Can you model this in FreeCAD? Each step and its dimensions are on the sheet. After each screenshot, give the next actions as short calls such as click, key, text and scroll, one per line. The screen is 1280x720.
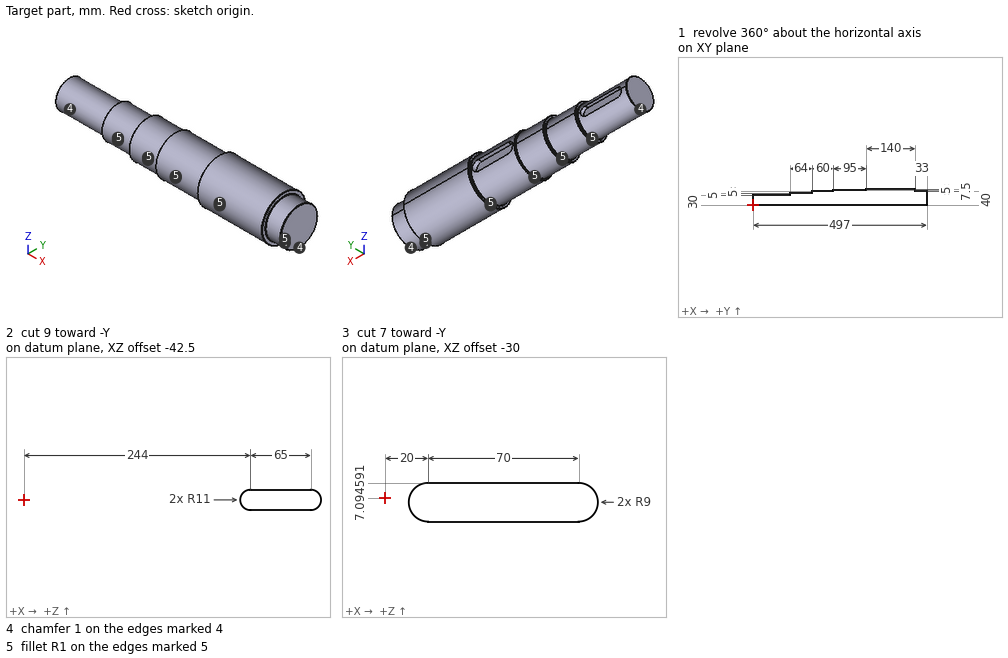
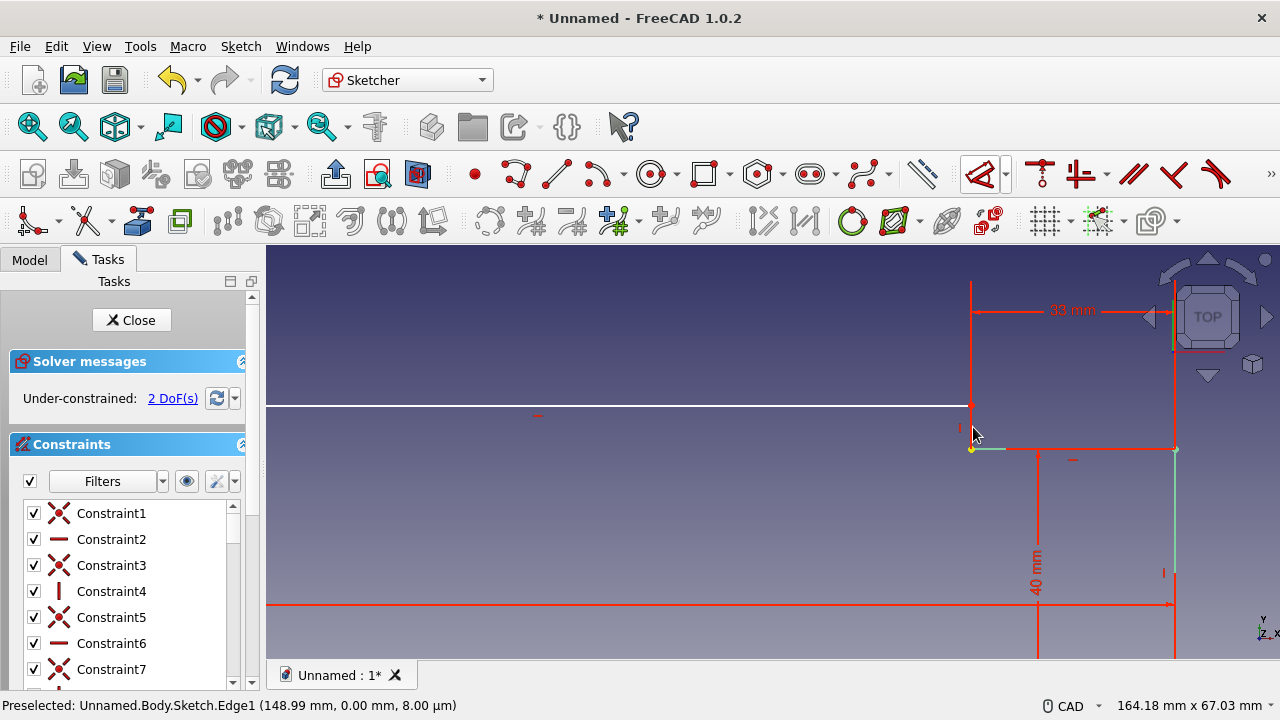
click(971, 427)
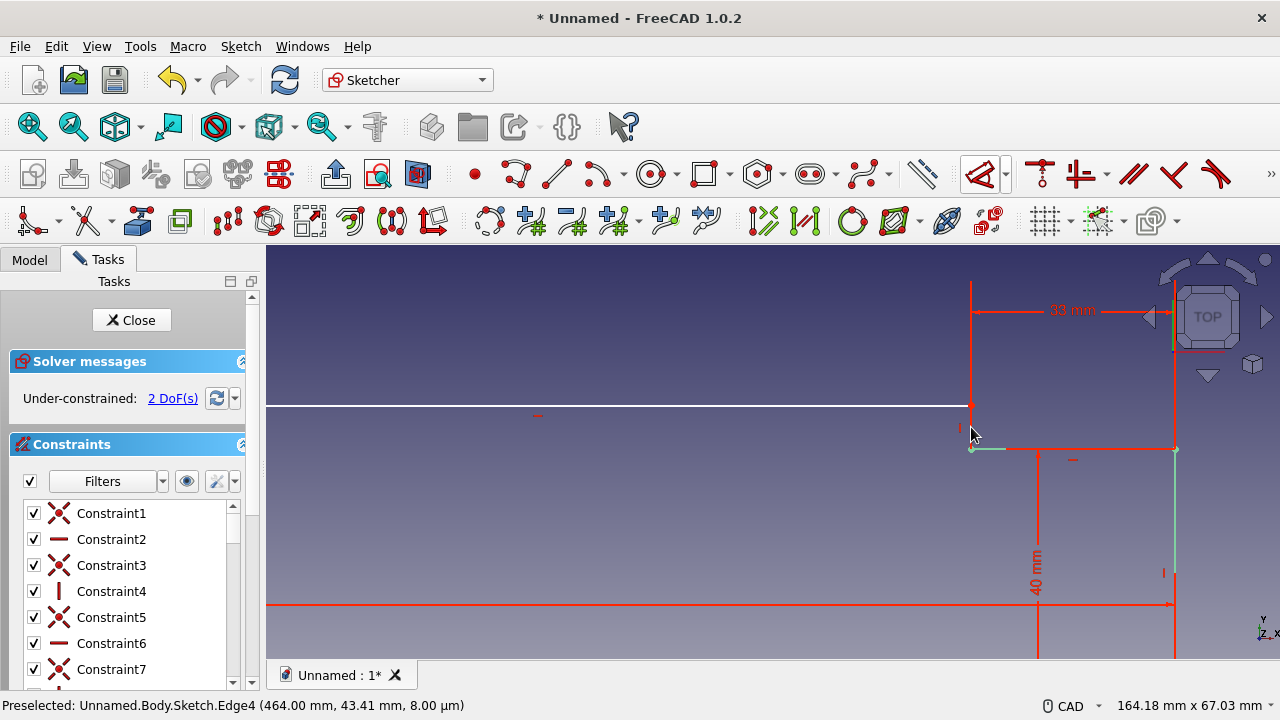
click(1006, 174)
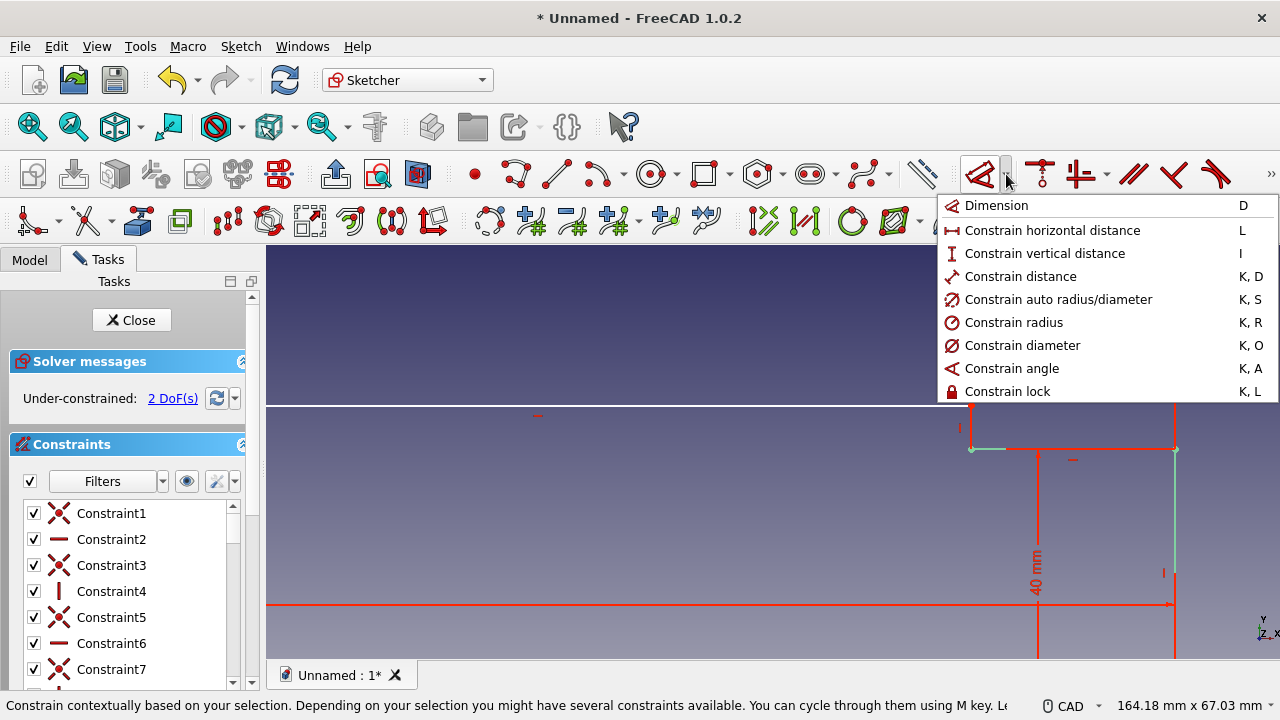
click(1108, 254)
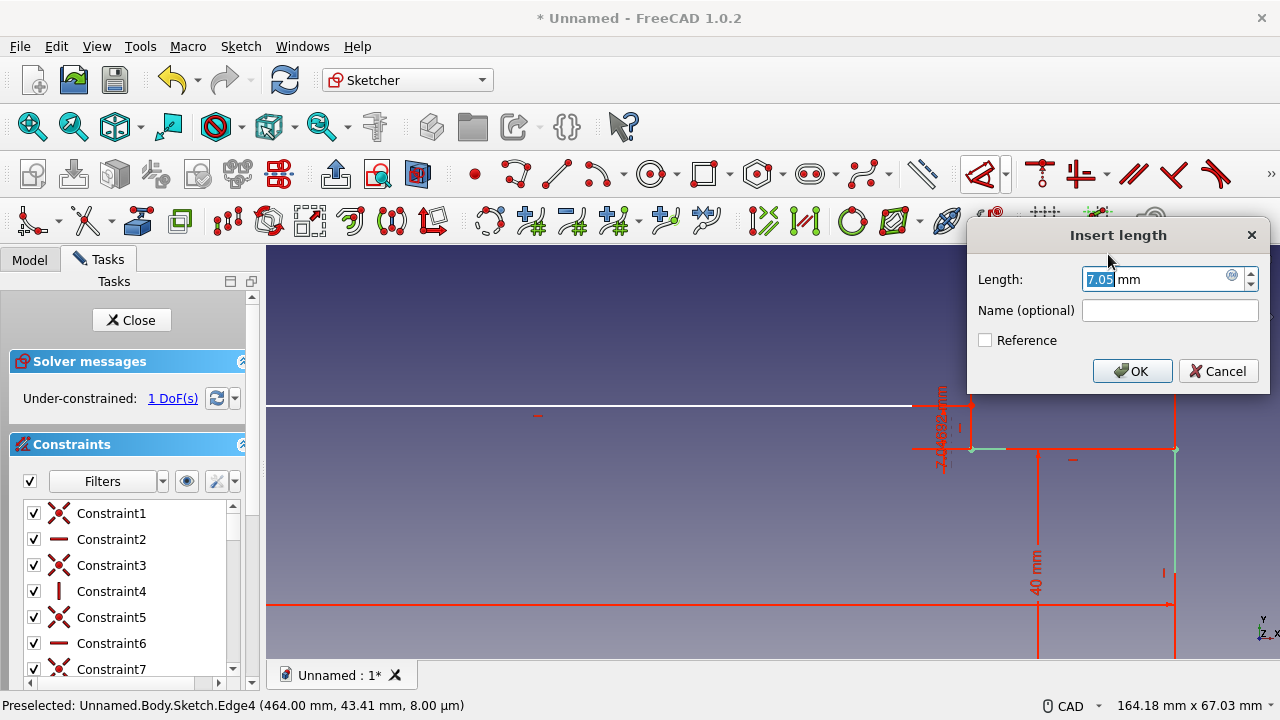
text(7.5)
key(Return)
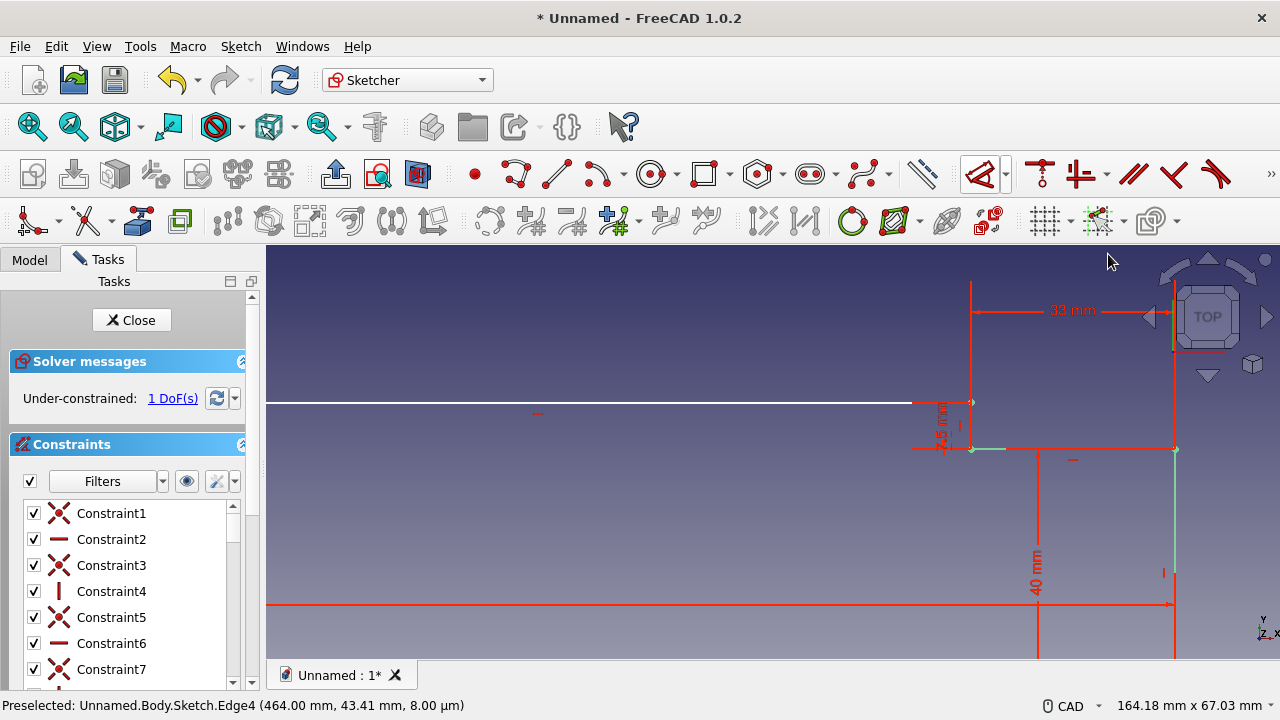
scroll(974, 427, down, 8)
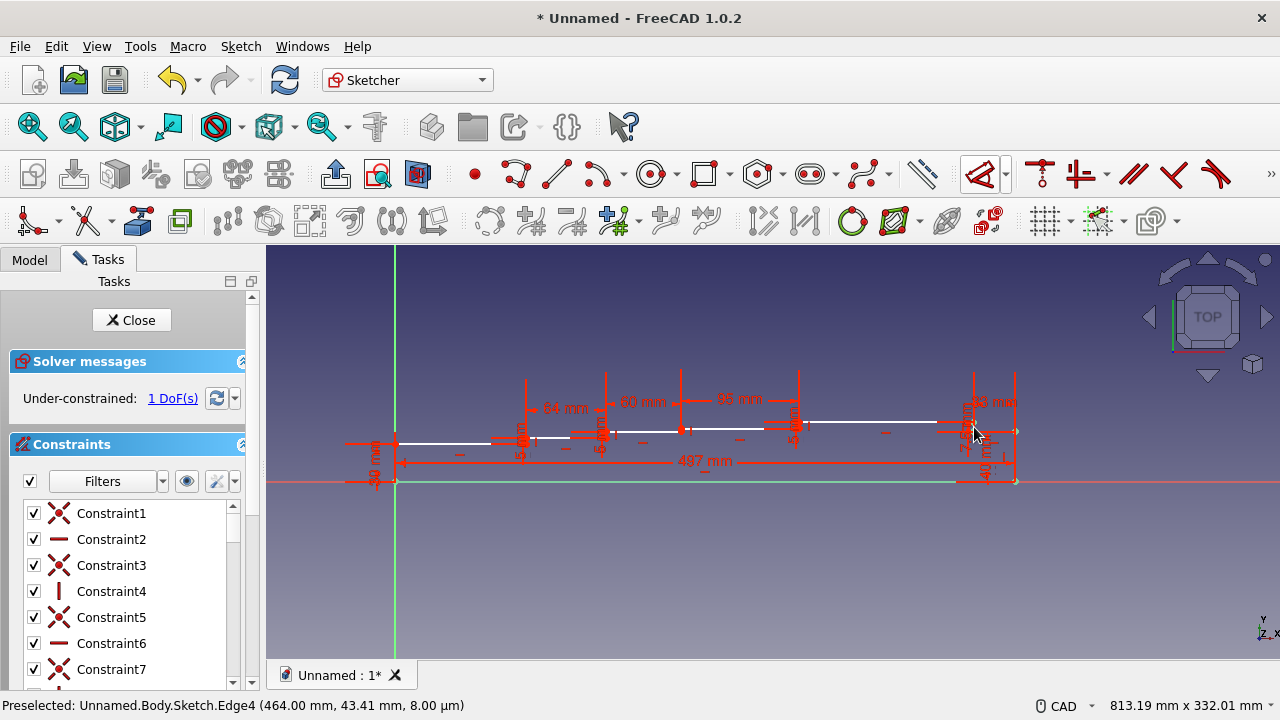
click(922, 422)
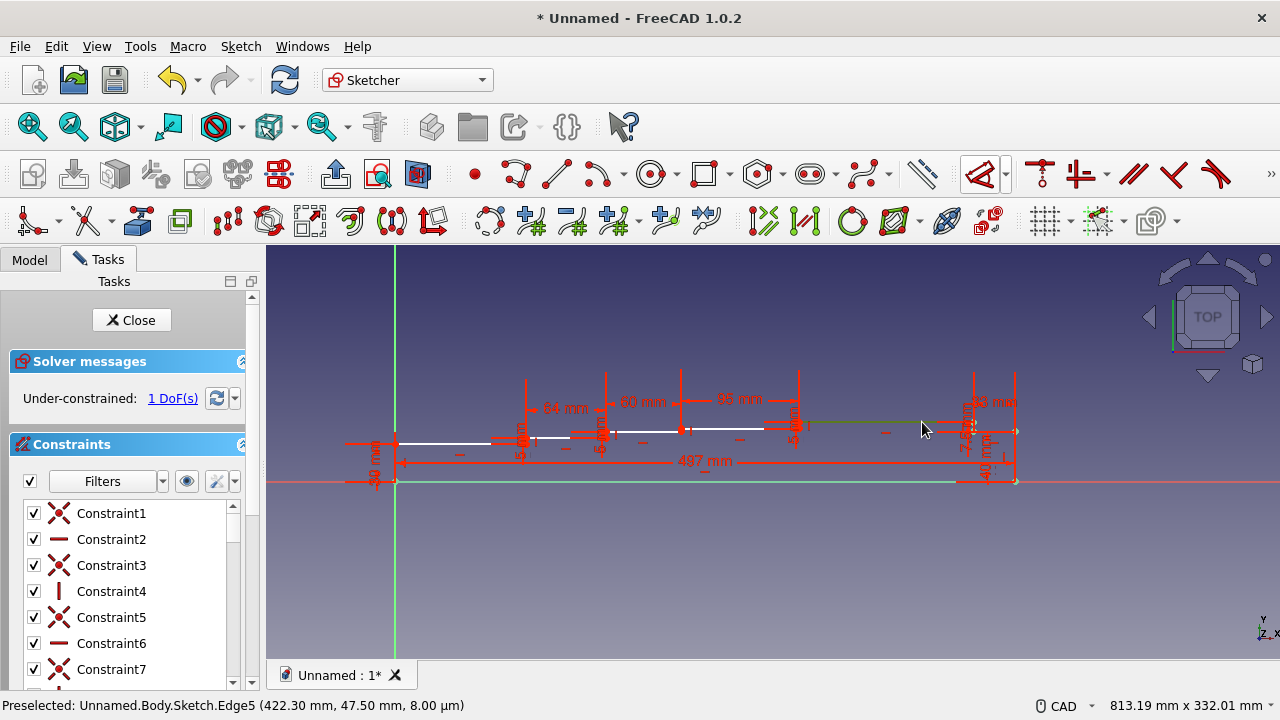
click(1006, 174)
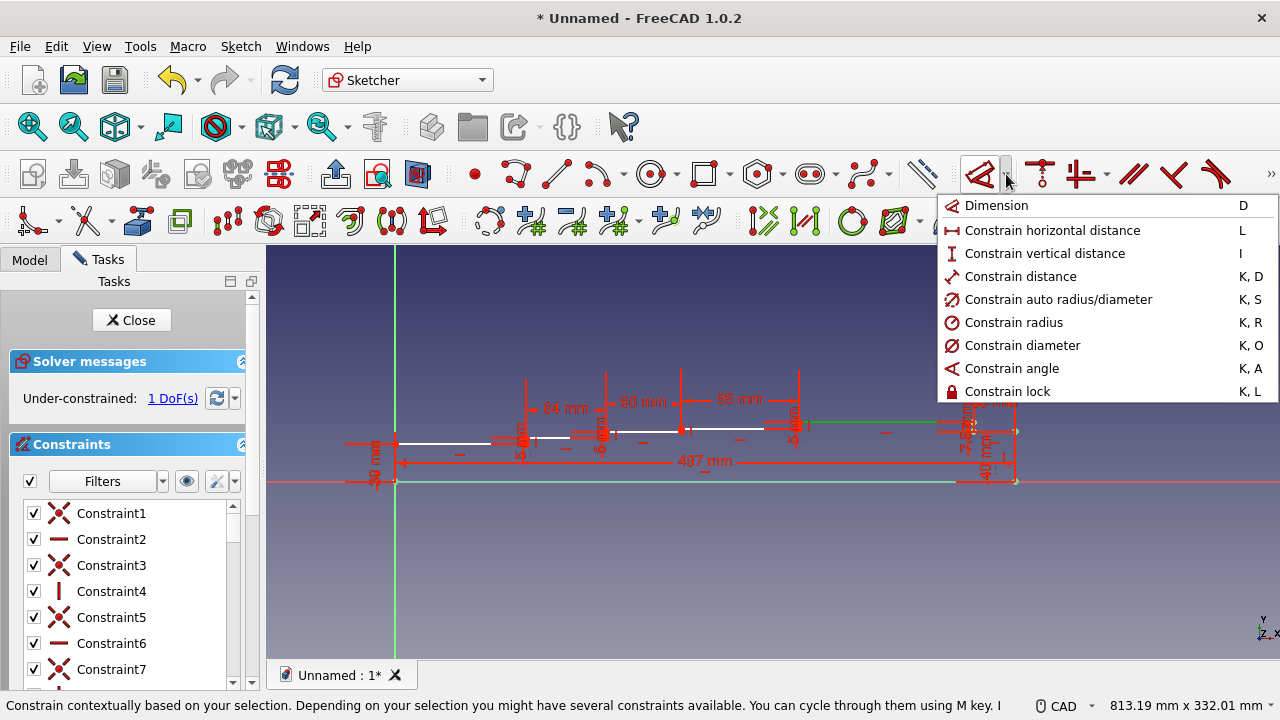
click(1108, 230)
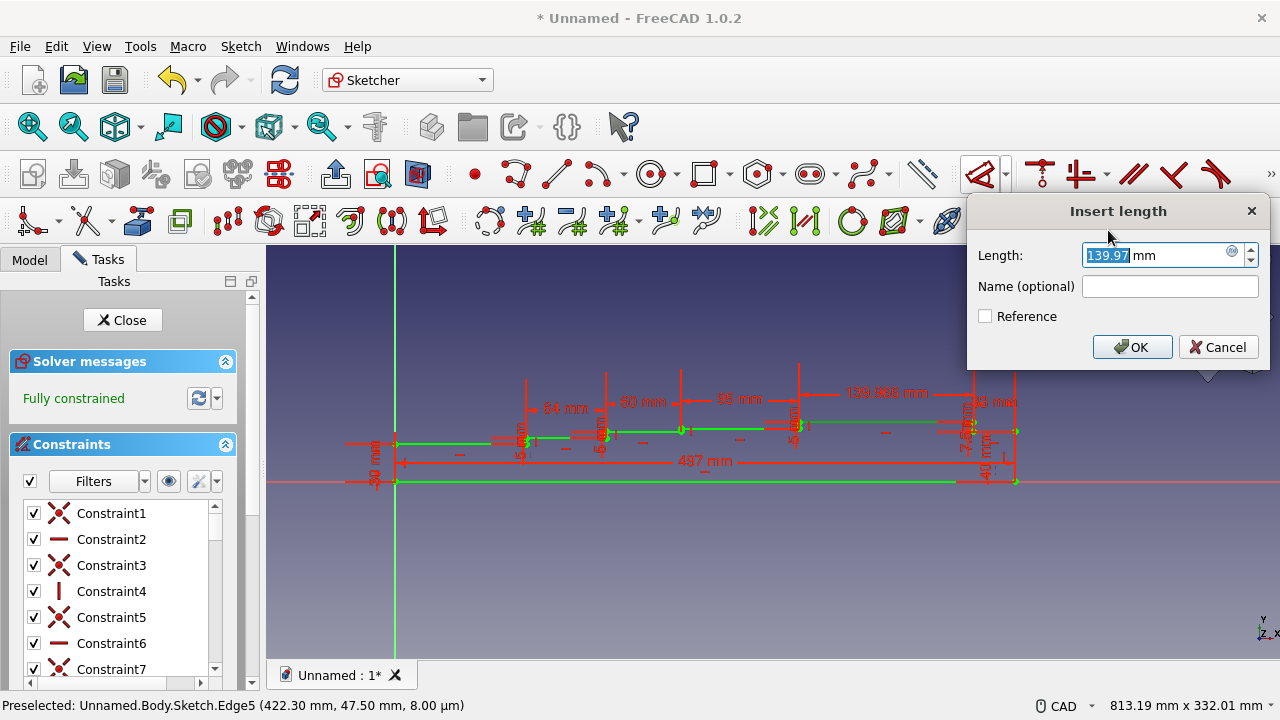
text(140)
key(Return)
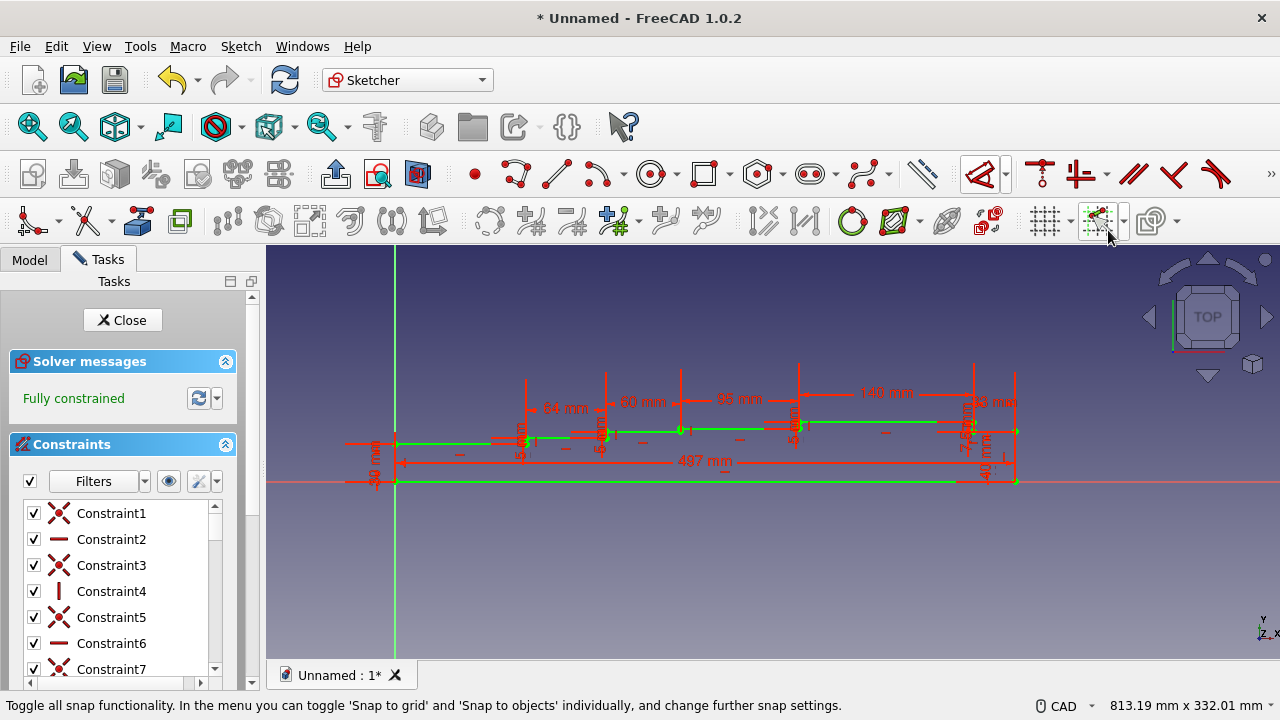
click(123, 320)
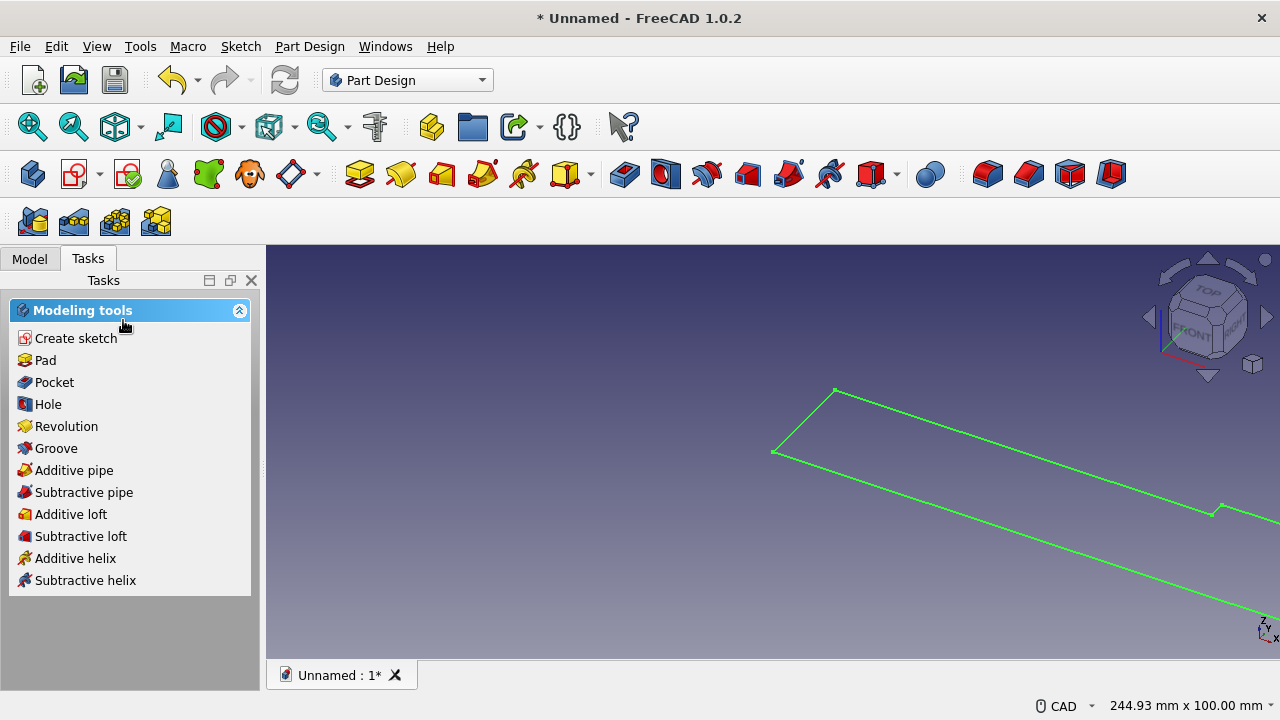
click(401, 174)